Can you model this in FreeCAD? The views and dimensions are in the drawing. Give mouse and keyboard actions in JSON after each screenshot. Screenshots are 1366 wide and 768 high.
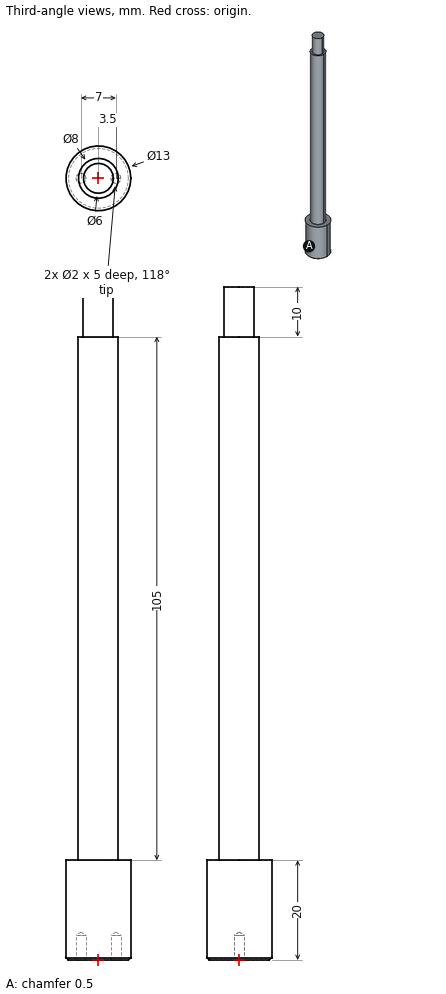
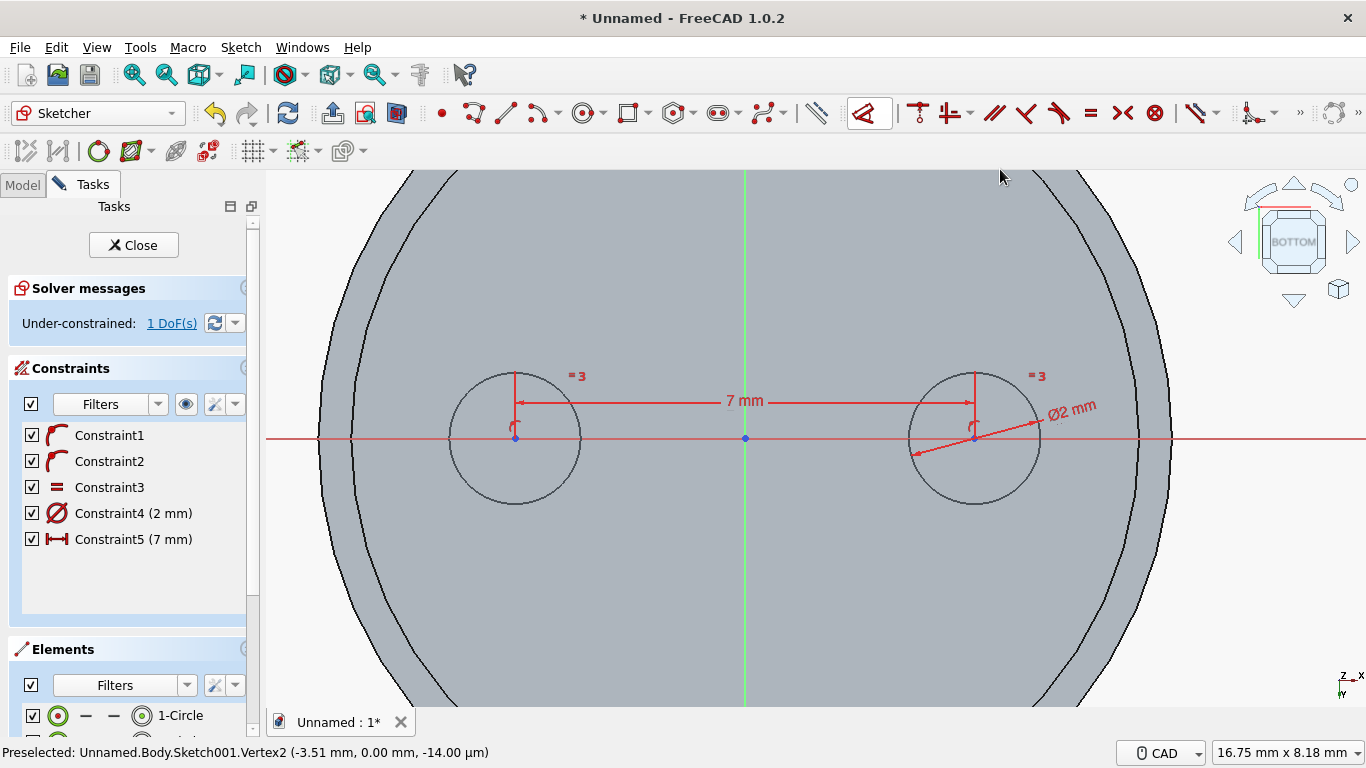
{"action": "left_click", "coordinate": [975, 438]}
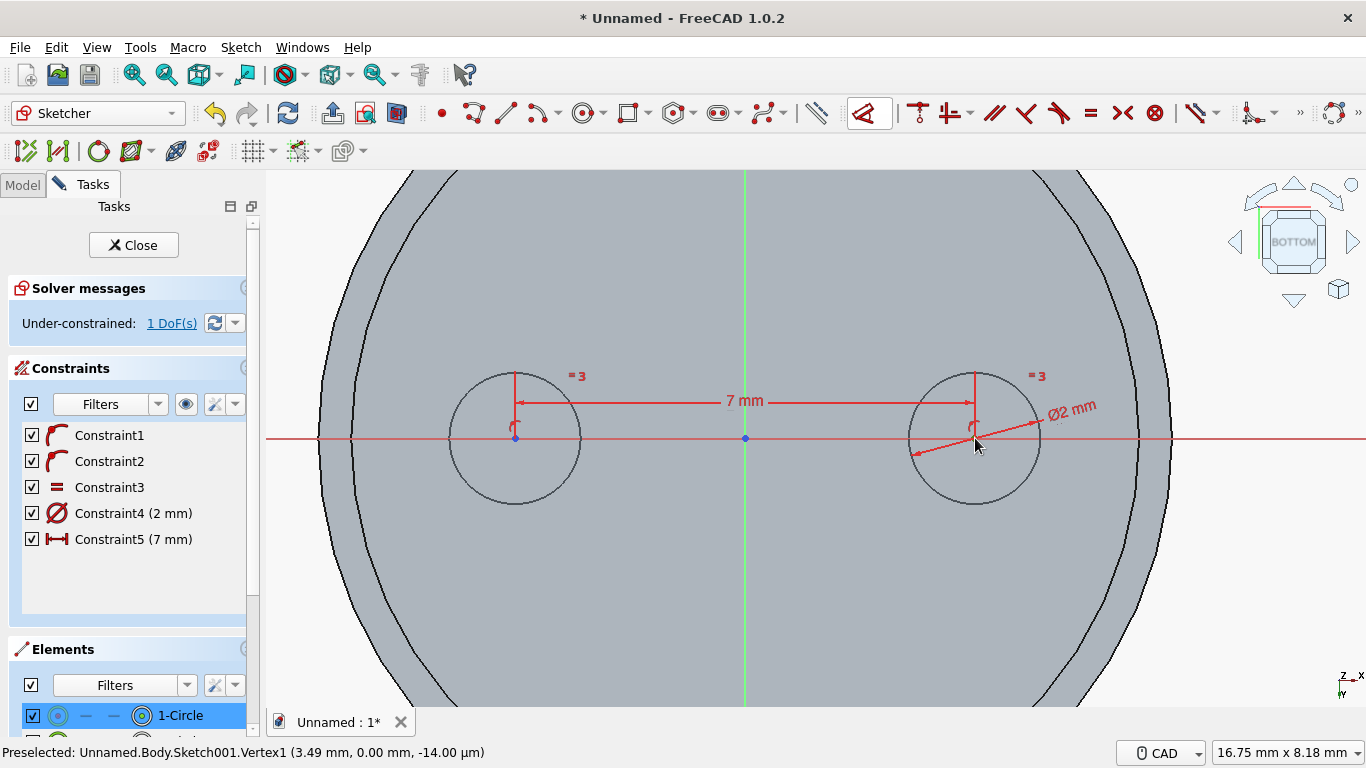
{"action": "left_click", "coordinate": [886, 114]}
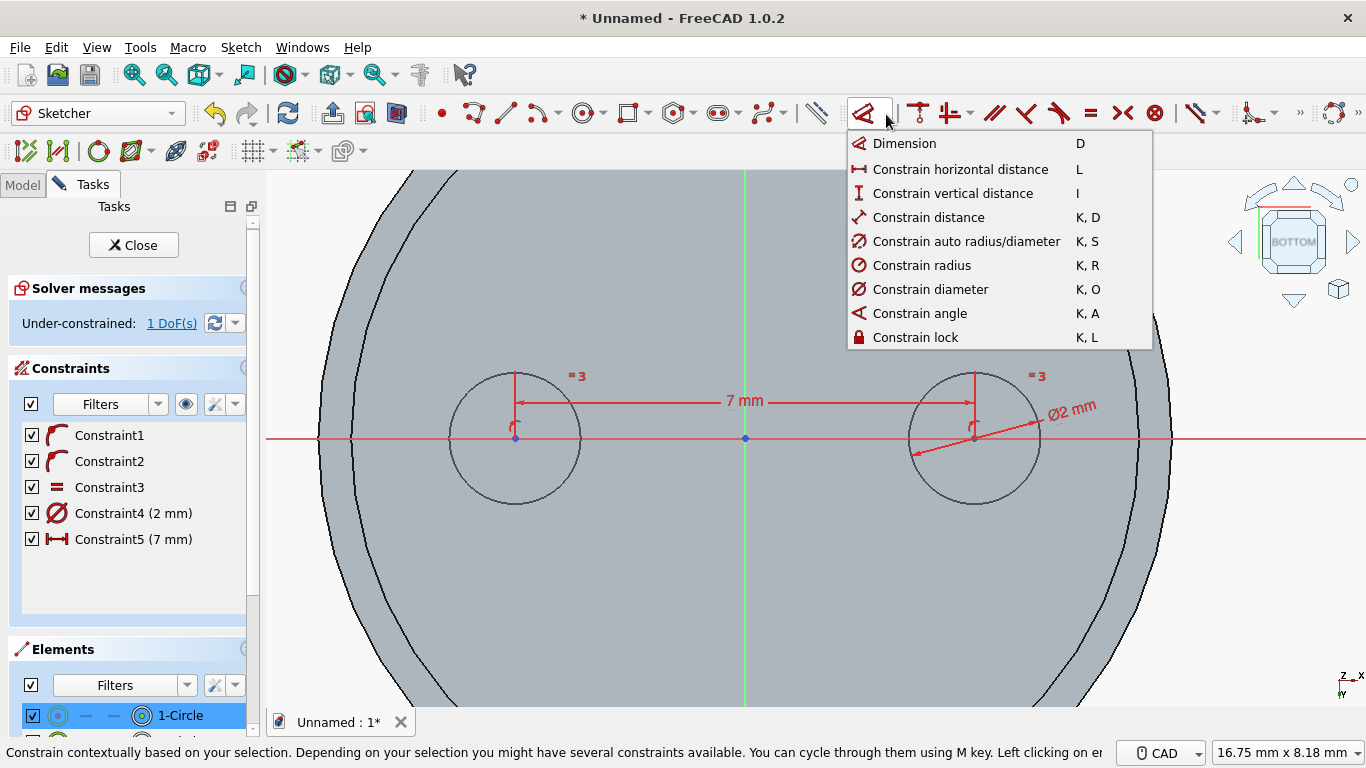
{"action": "left_click", "coordinate": [1000, 169]}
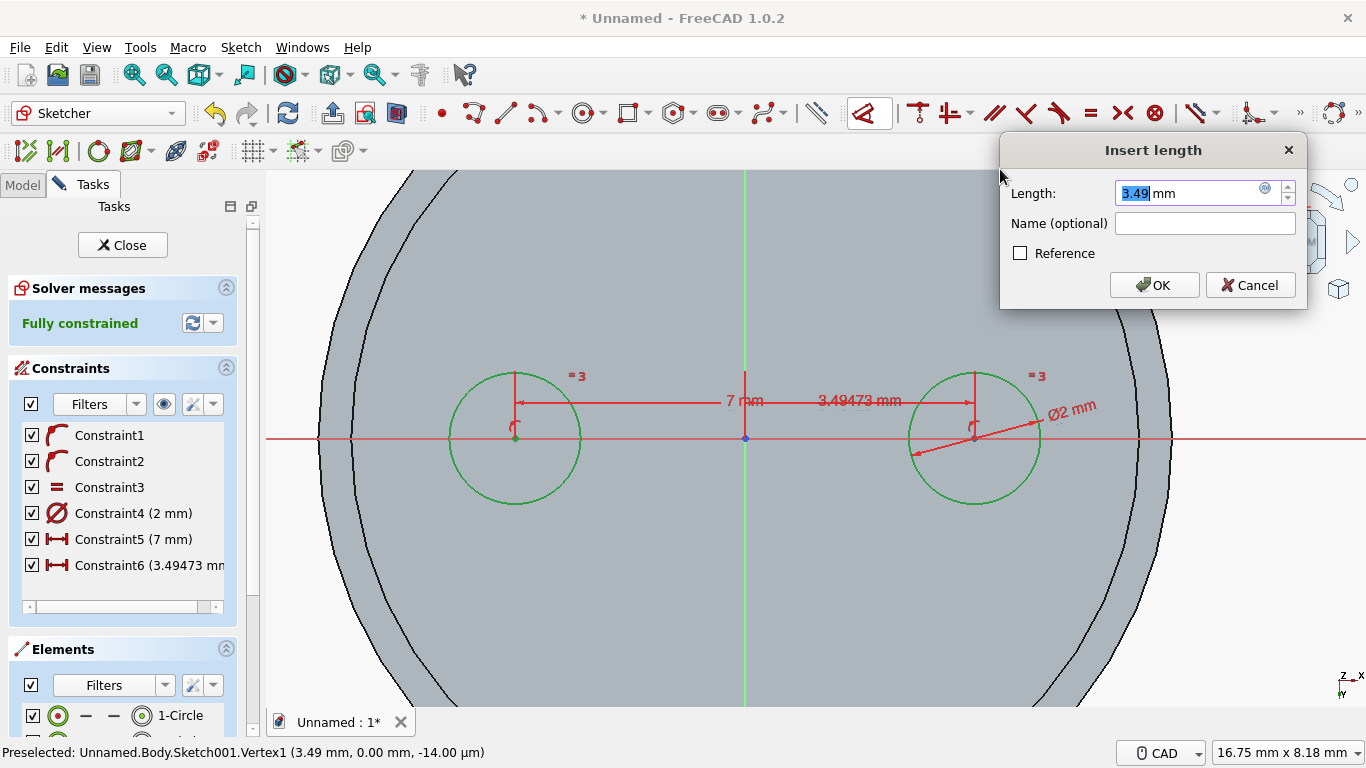
{"action": "type", "text": "3.5"}
{"action": "key", "text": "Return"}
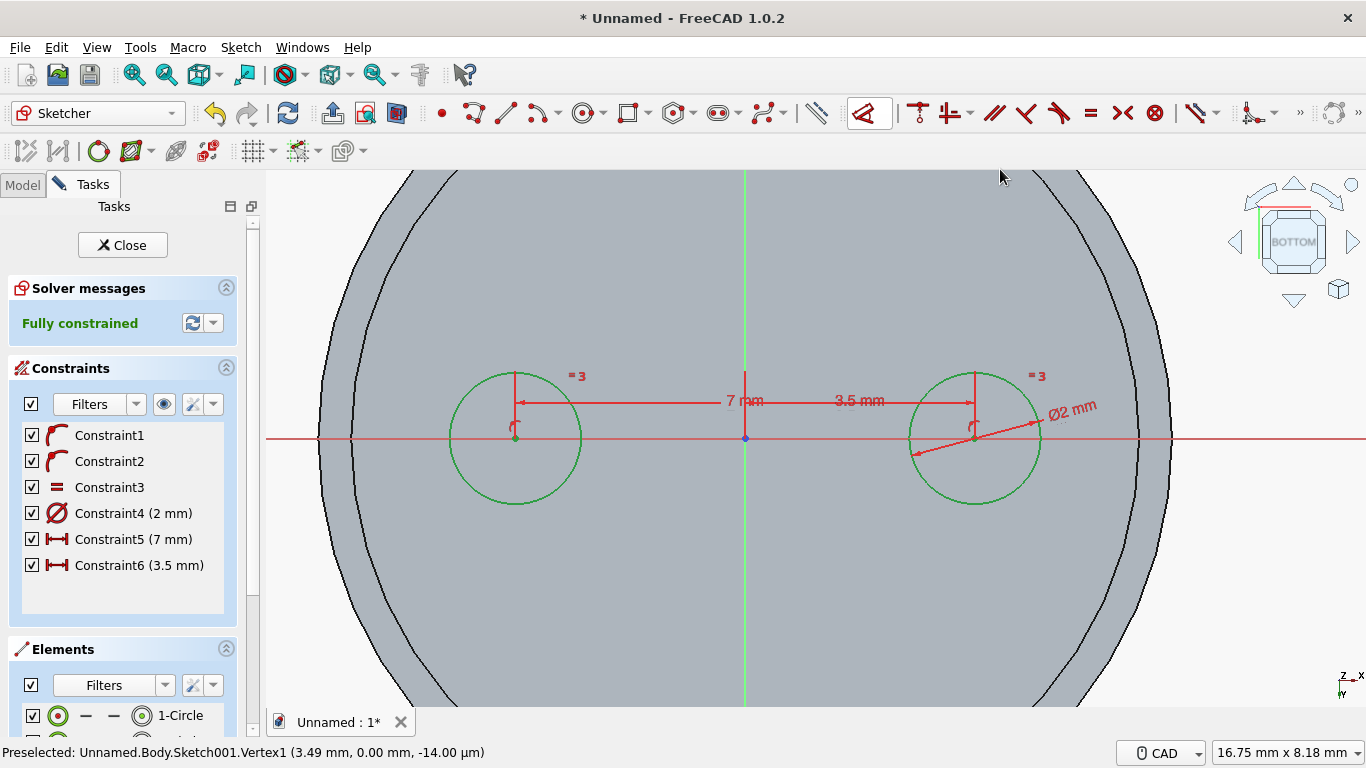
{"action": "left_click", "coordinate": [123, 245]}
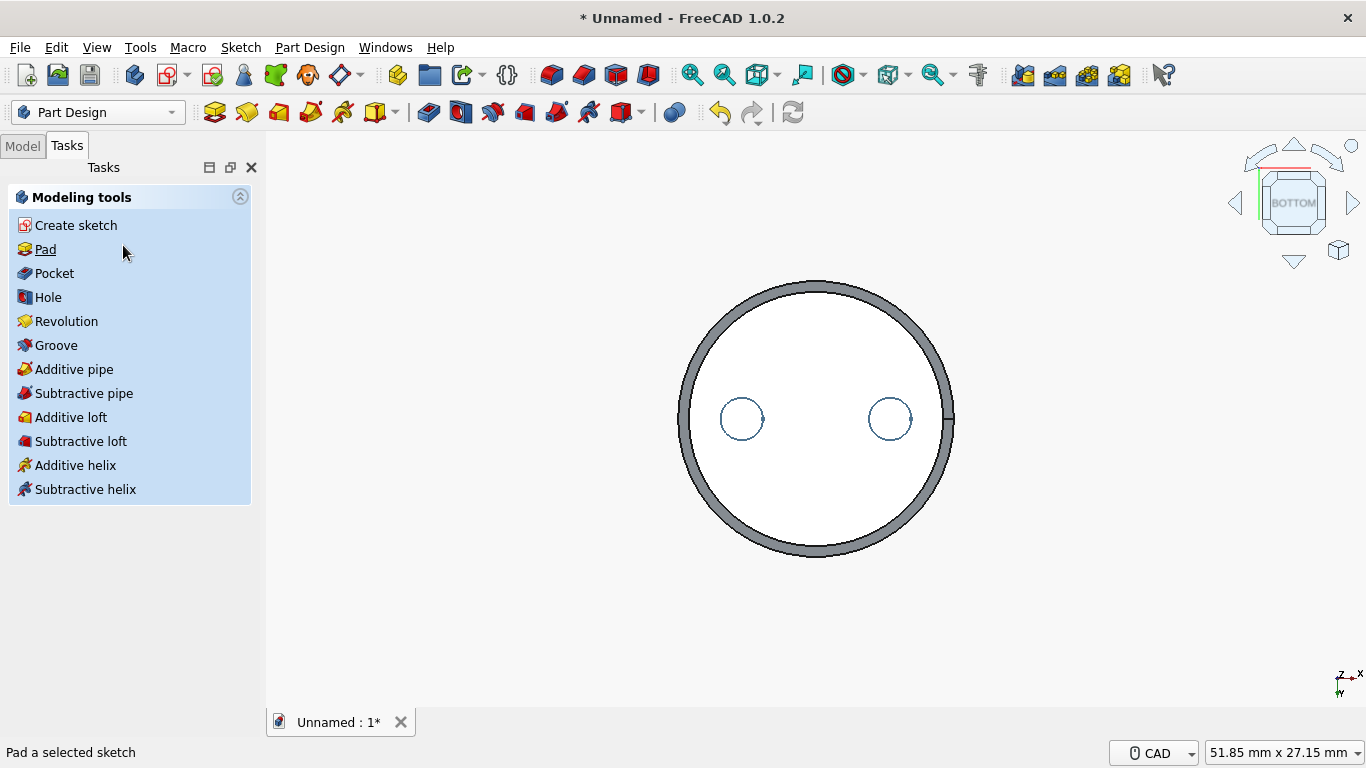
{"action": "left_click", "coordinate": [462, 112]}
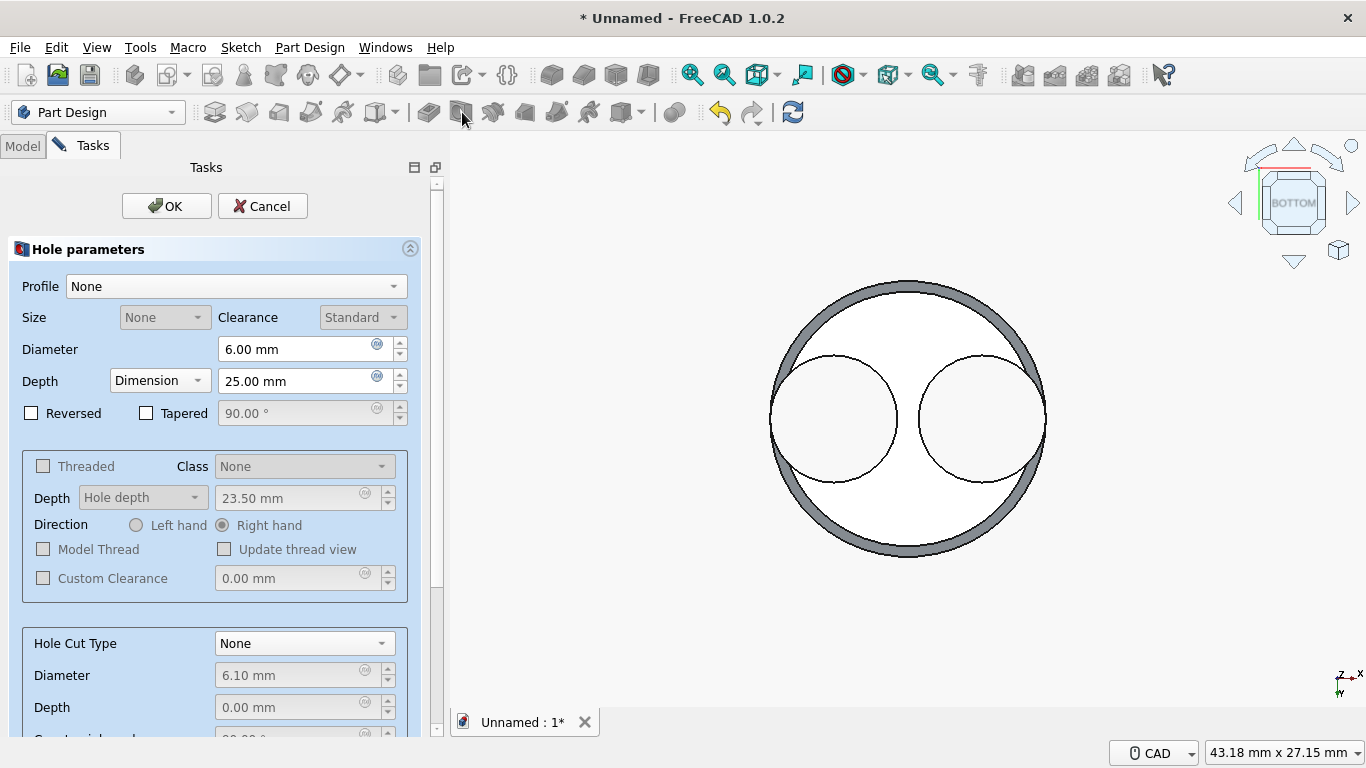
{"action": "triple_click", "coordinate": [305, 349]}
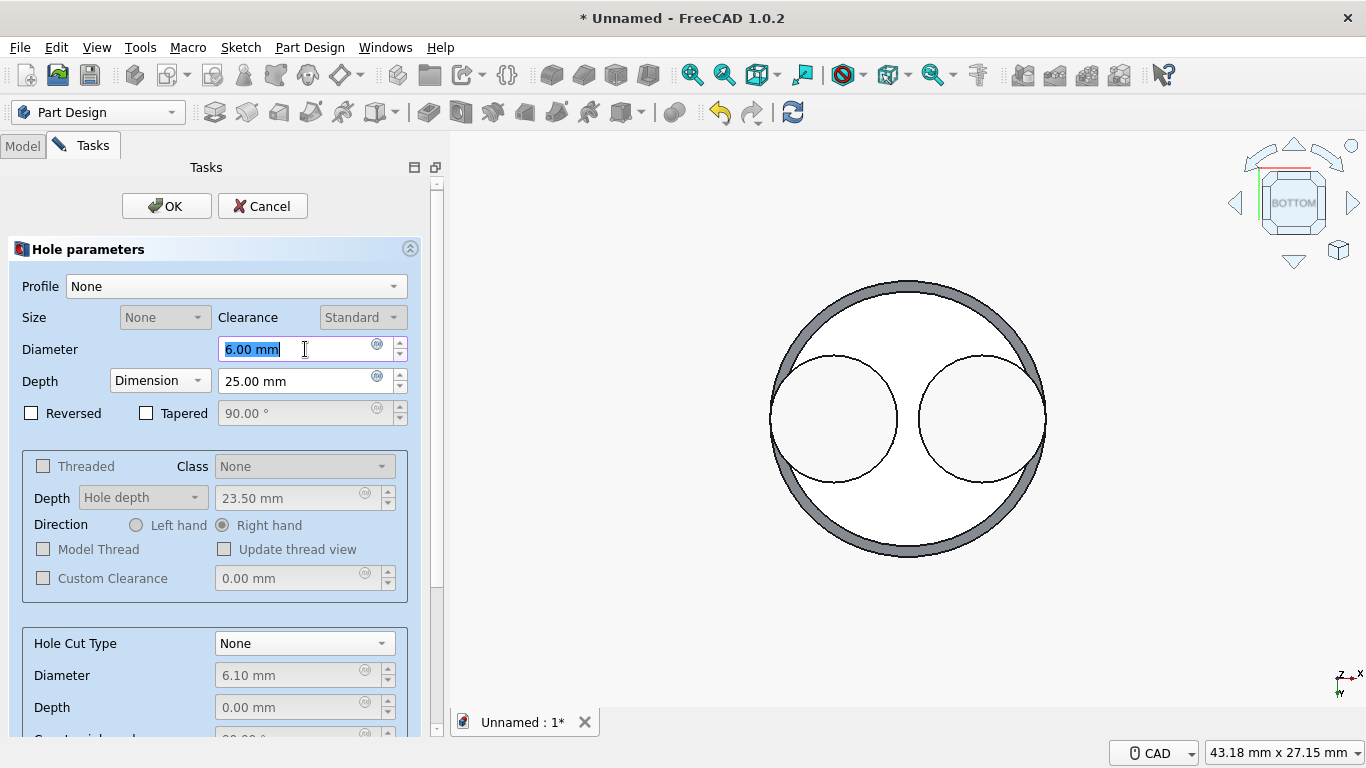
{"action": "type", "text": "2"}
{"action": "key", "text": "Tab"}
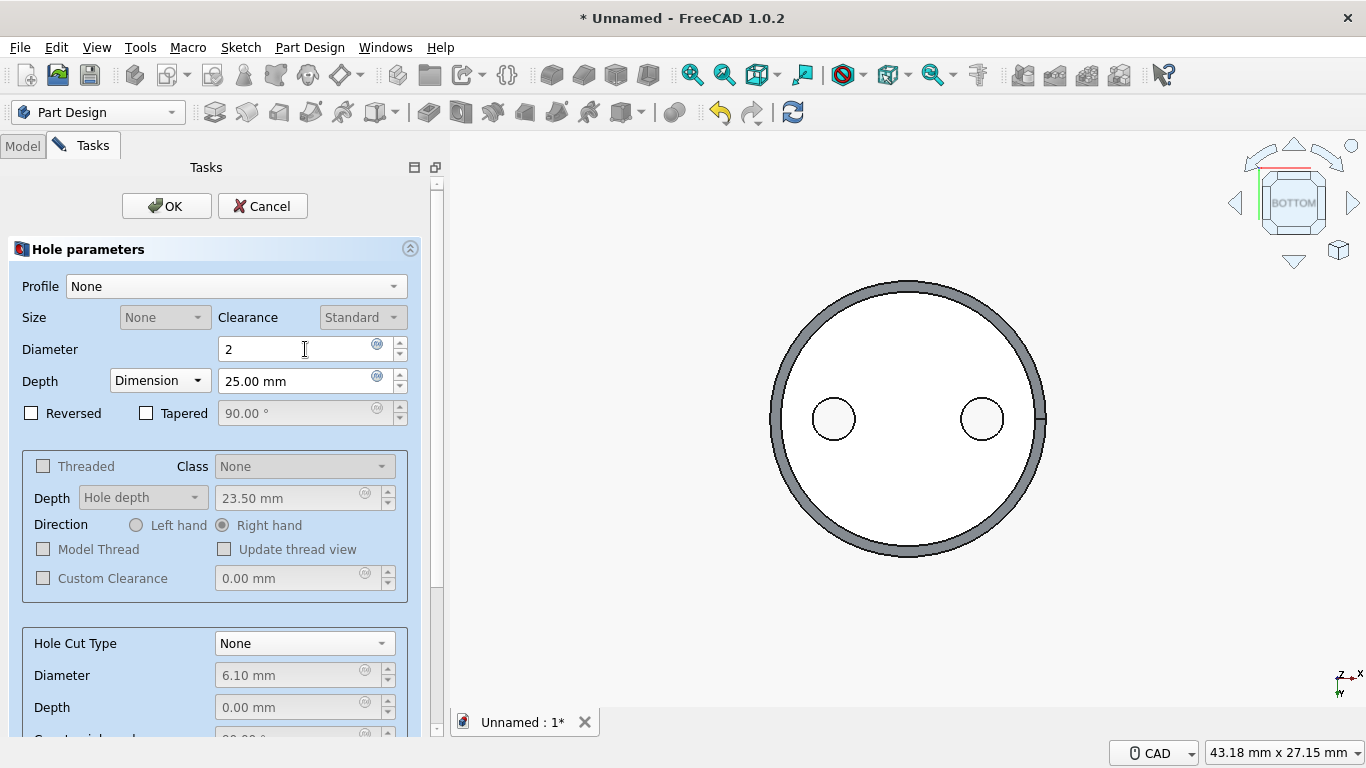
{"action": "triple_click", "coordinate": [305, 381]}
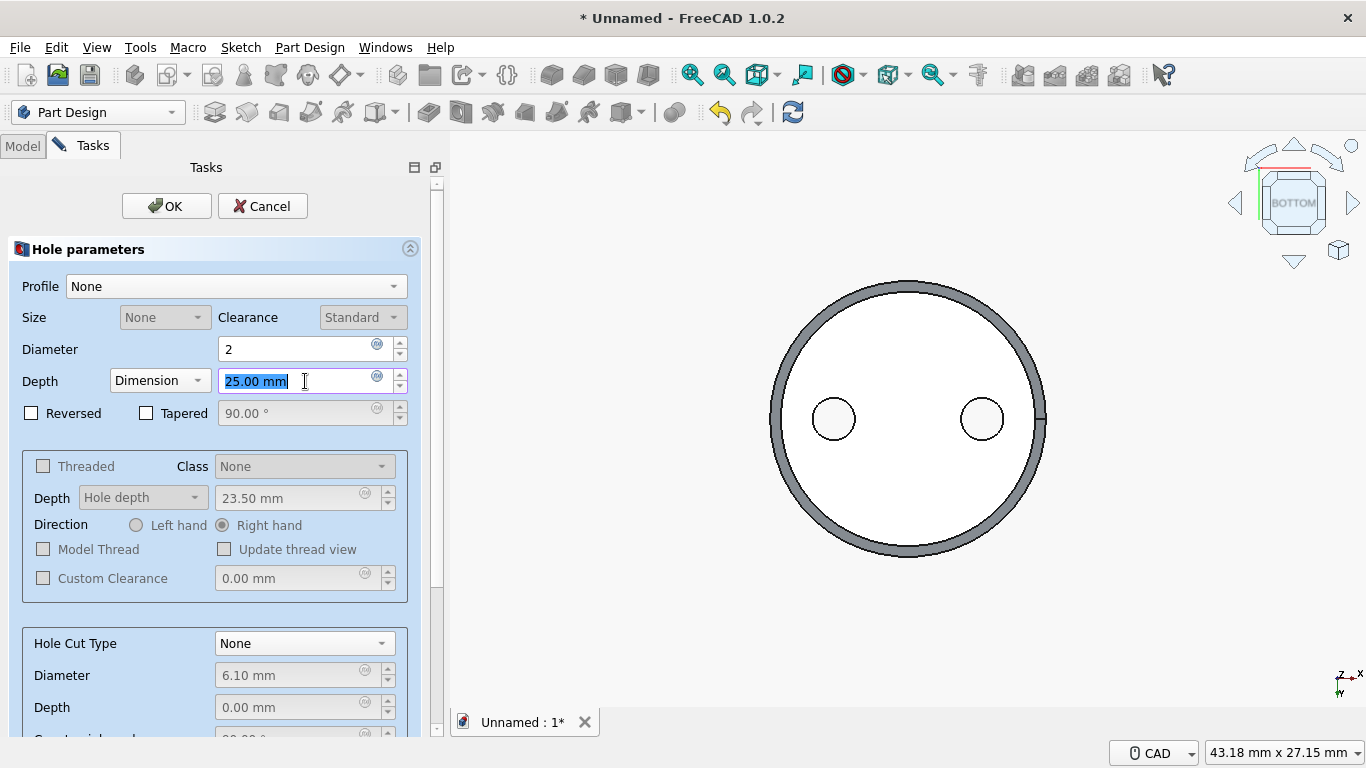
{"action": "type", "text": "5"}
{"action": "key", "text": "Tab"}